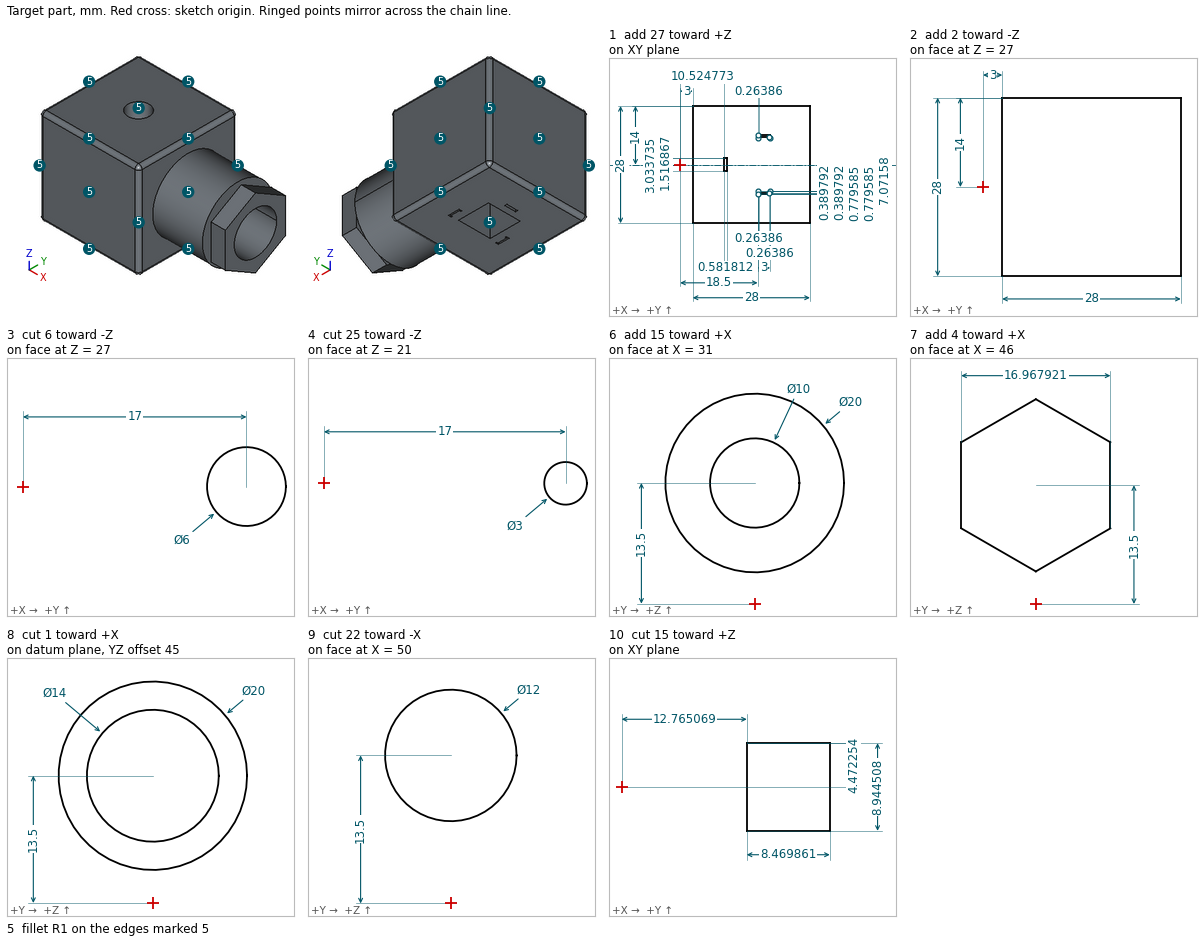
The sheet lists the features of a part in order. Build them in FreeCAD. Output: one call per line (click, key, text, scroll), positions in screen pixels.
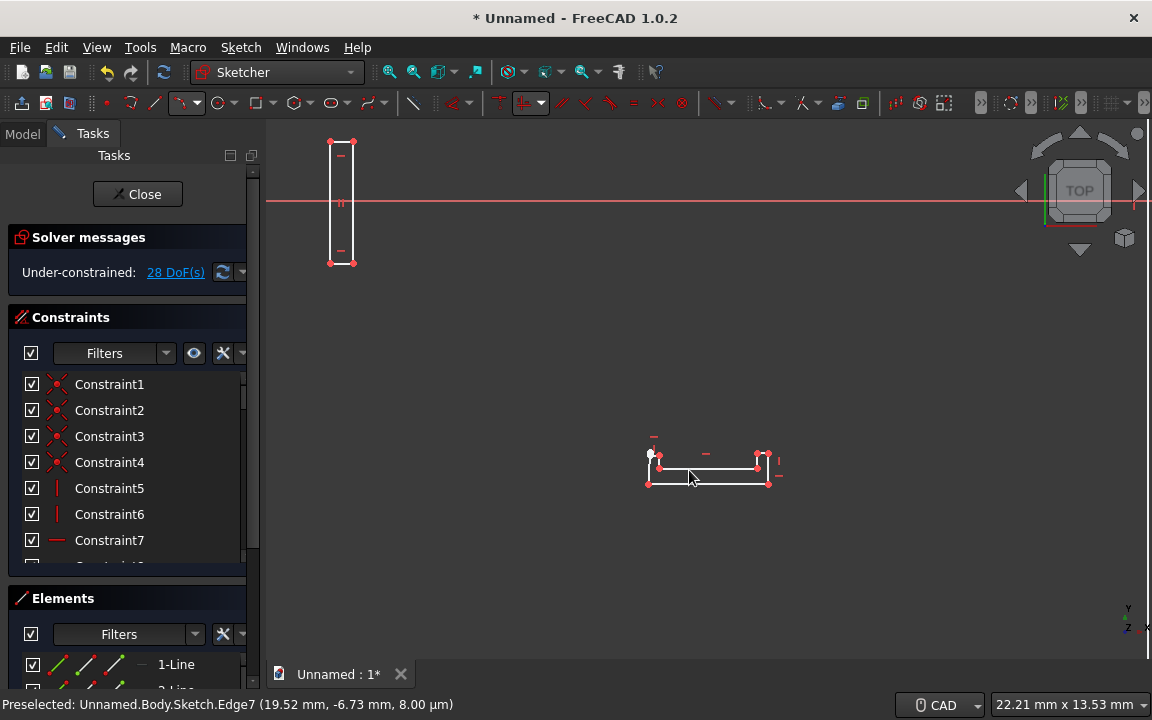
scroll(649, 475, up, 2)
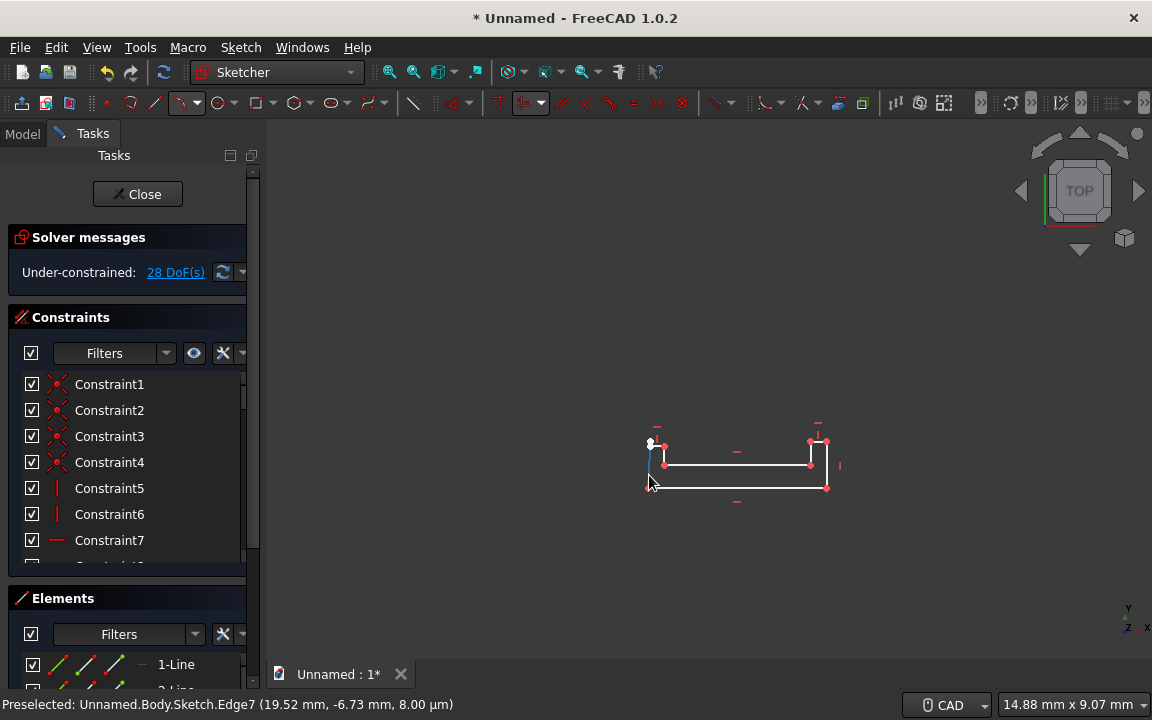
click(649, 474)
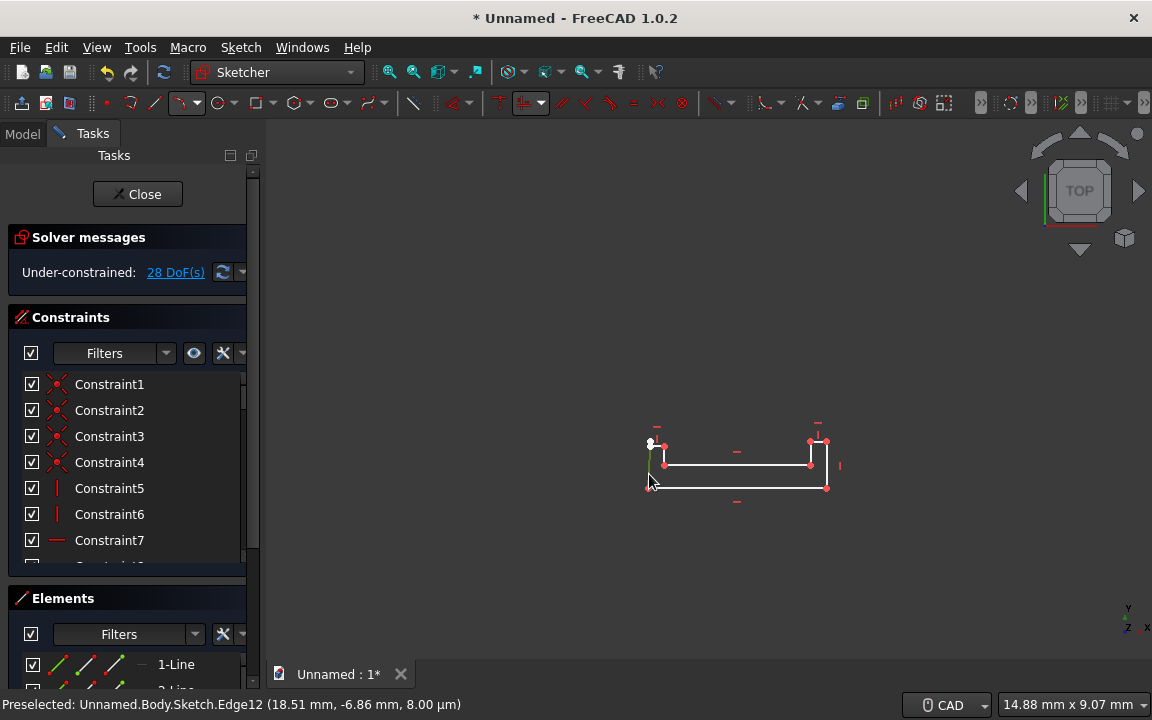
click(544, 104)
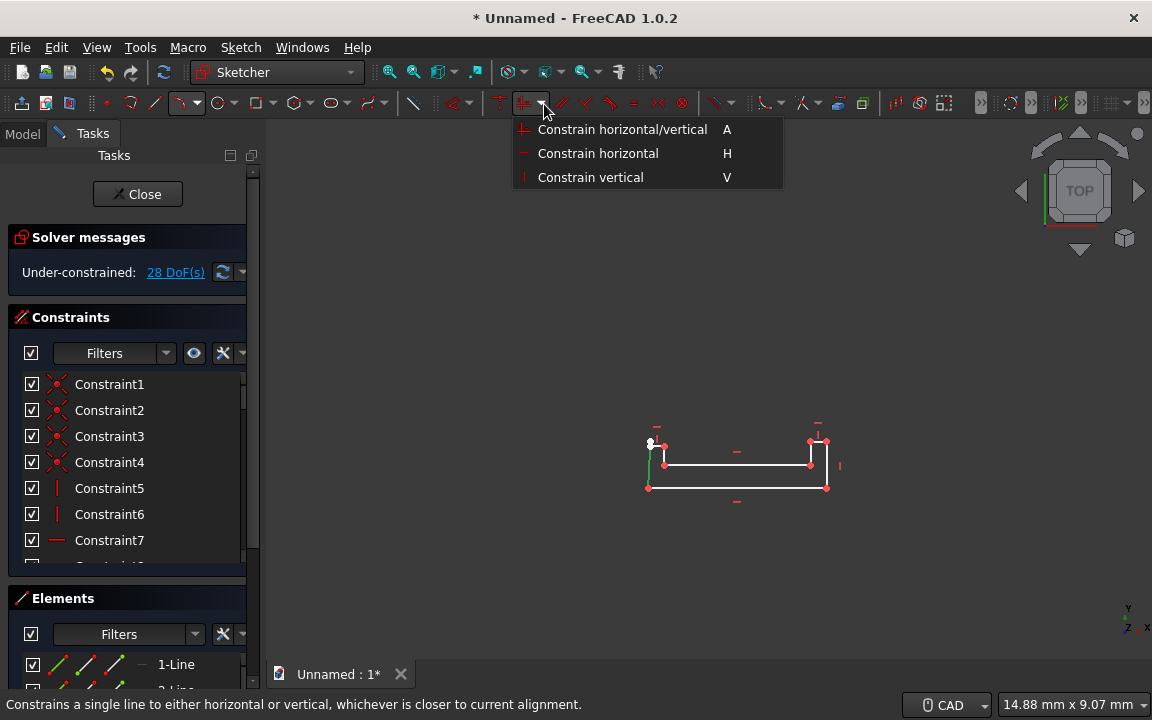
click(648, 177)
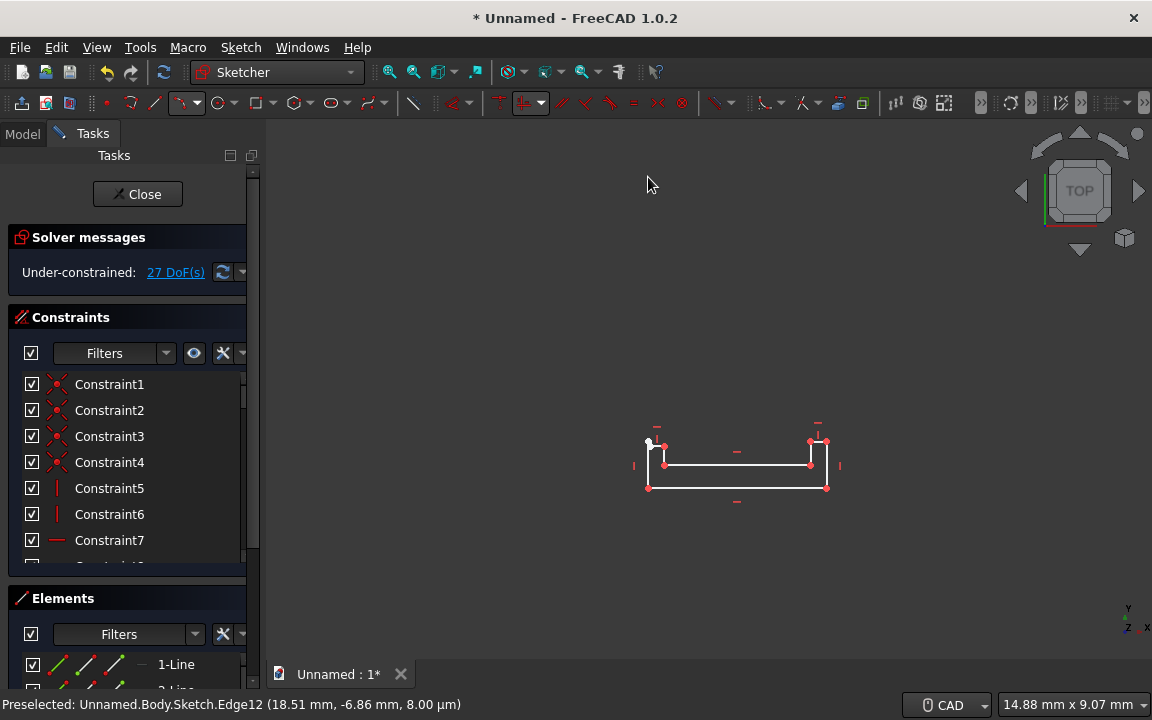
scroll(684, 471, down, 8)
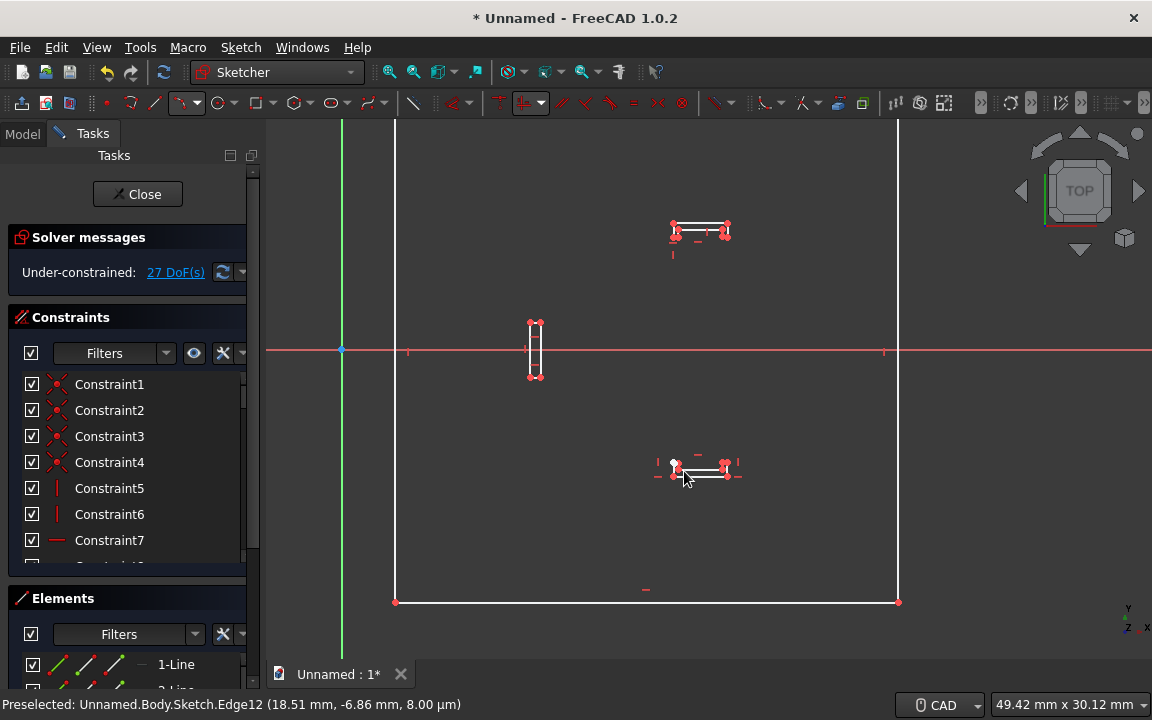
scroll(712, 314, up, 11)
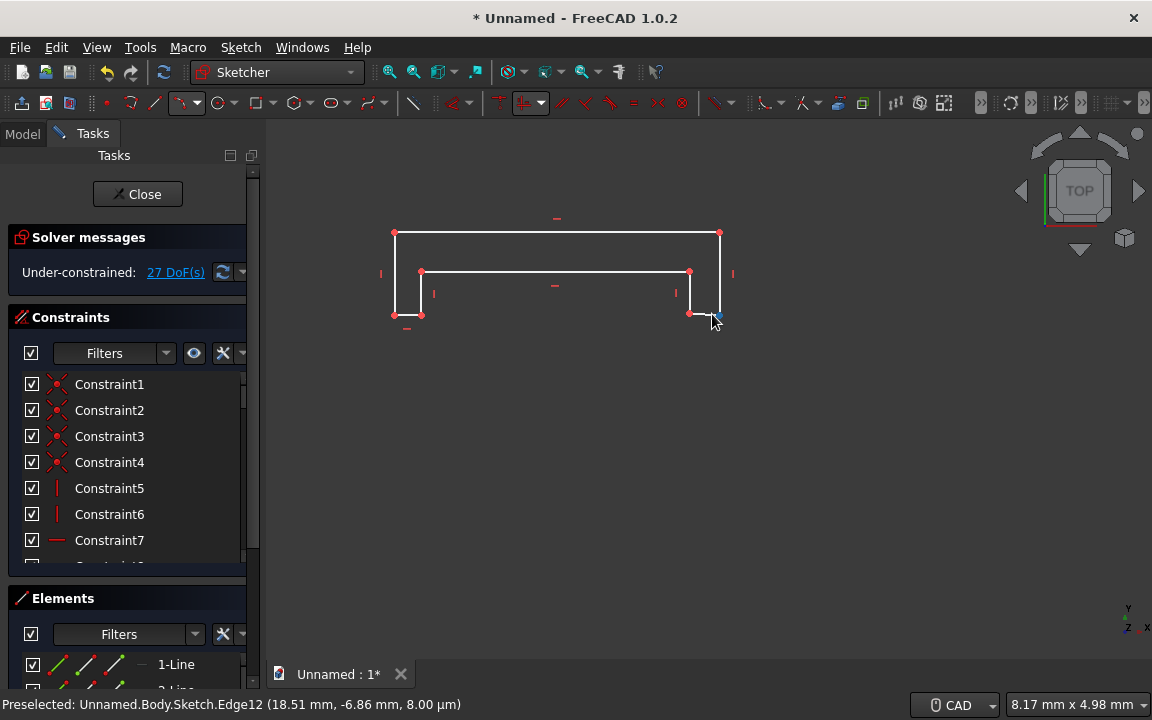
click(705, 314)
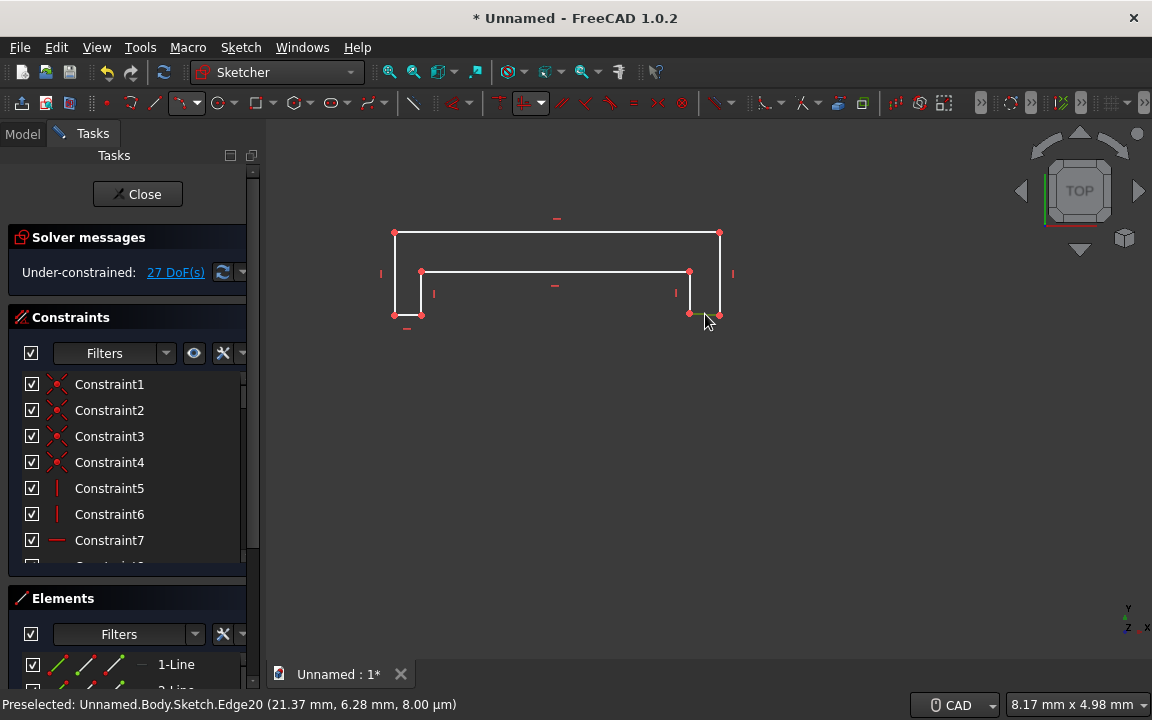
click(544, 104)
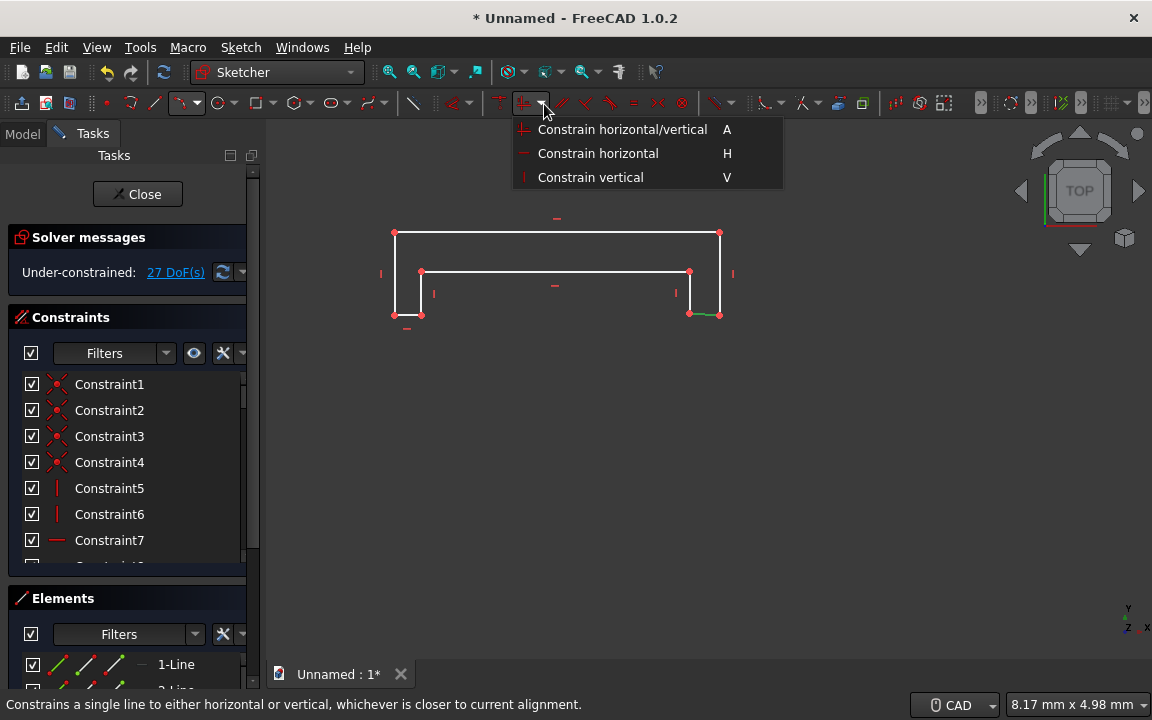
click(648, 153)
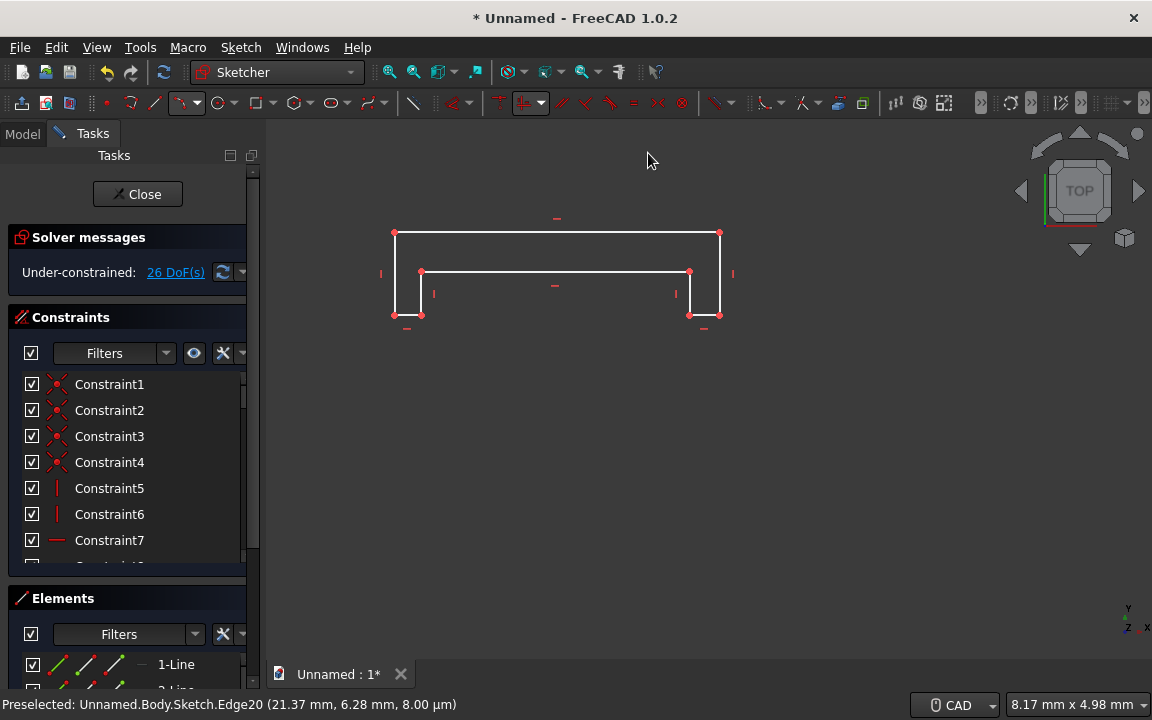
scroll(712, 313, down, 11)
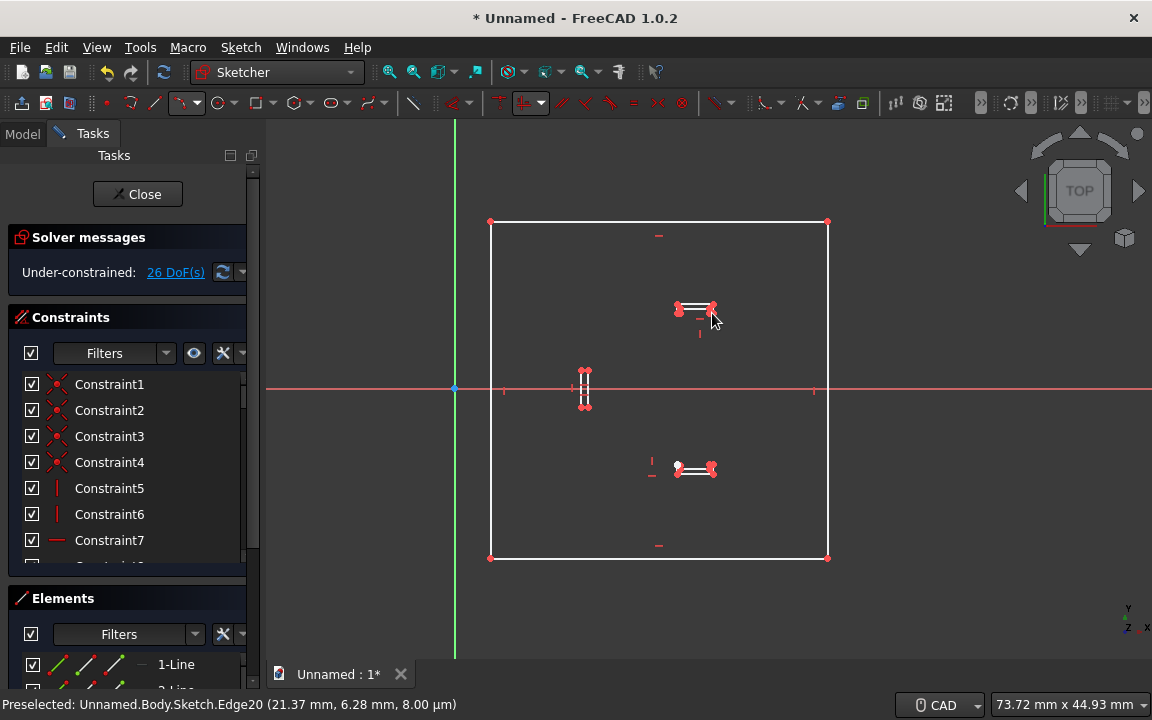
scroll(678, 466, up, 8)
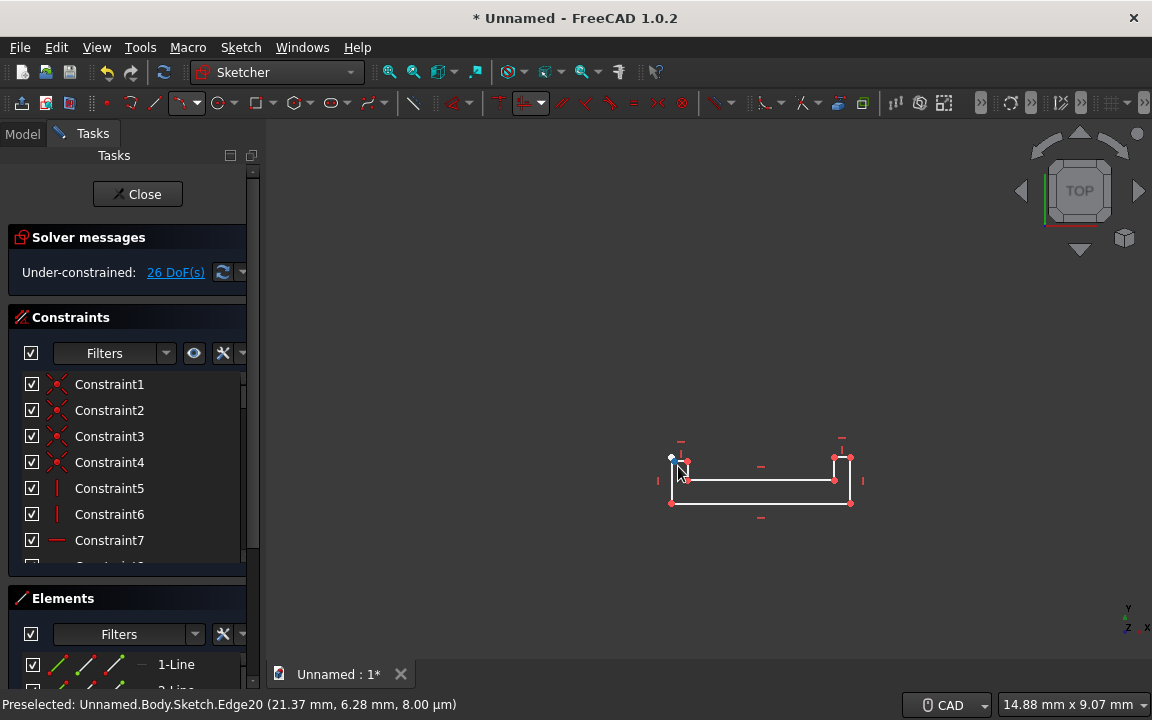
click(674, 461)